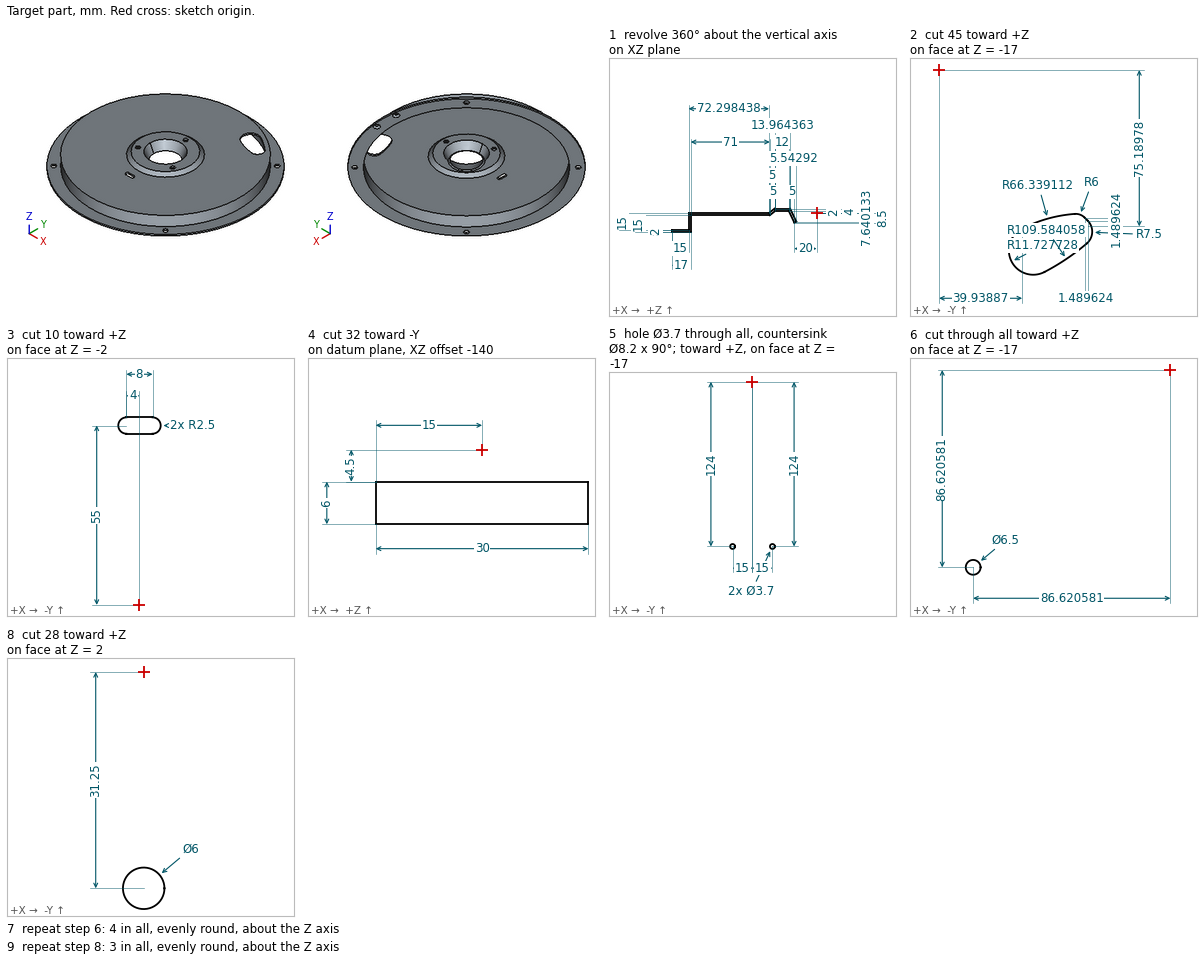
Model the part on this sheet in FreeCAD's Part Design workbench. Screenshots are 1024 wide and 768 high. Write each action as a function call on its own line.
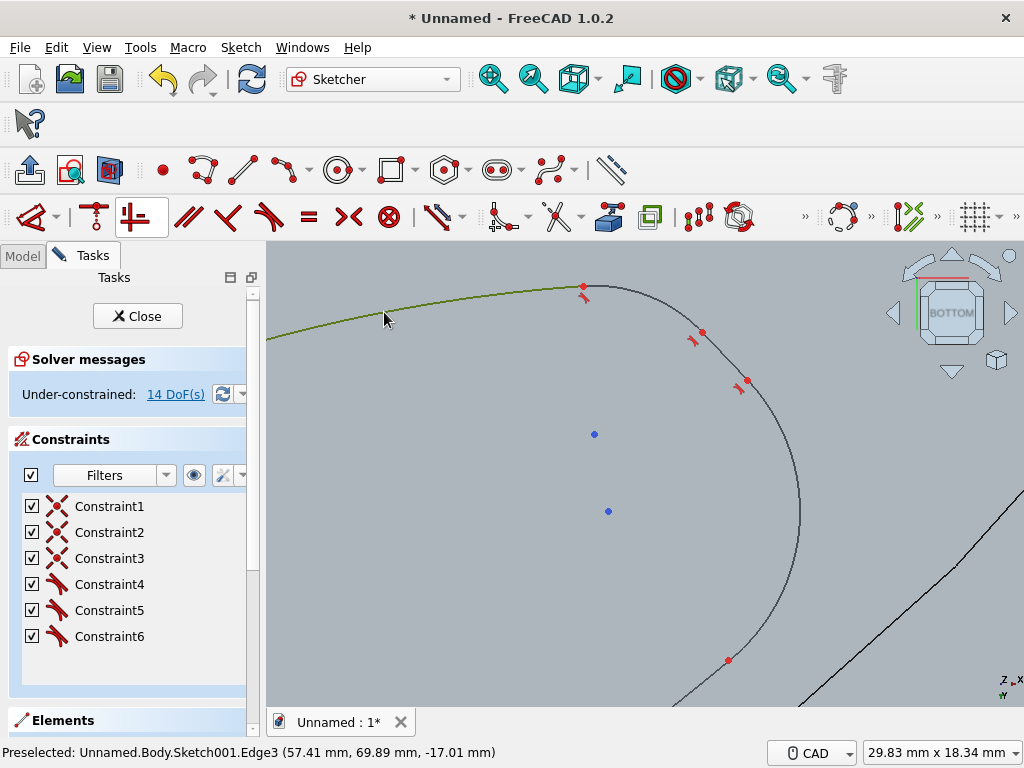
scroll(735, 372, down, 5)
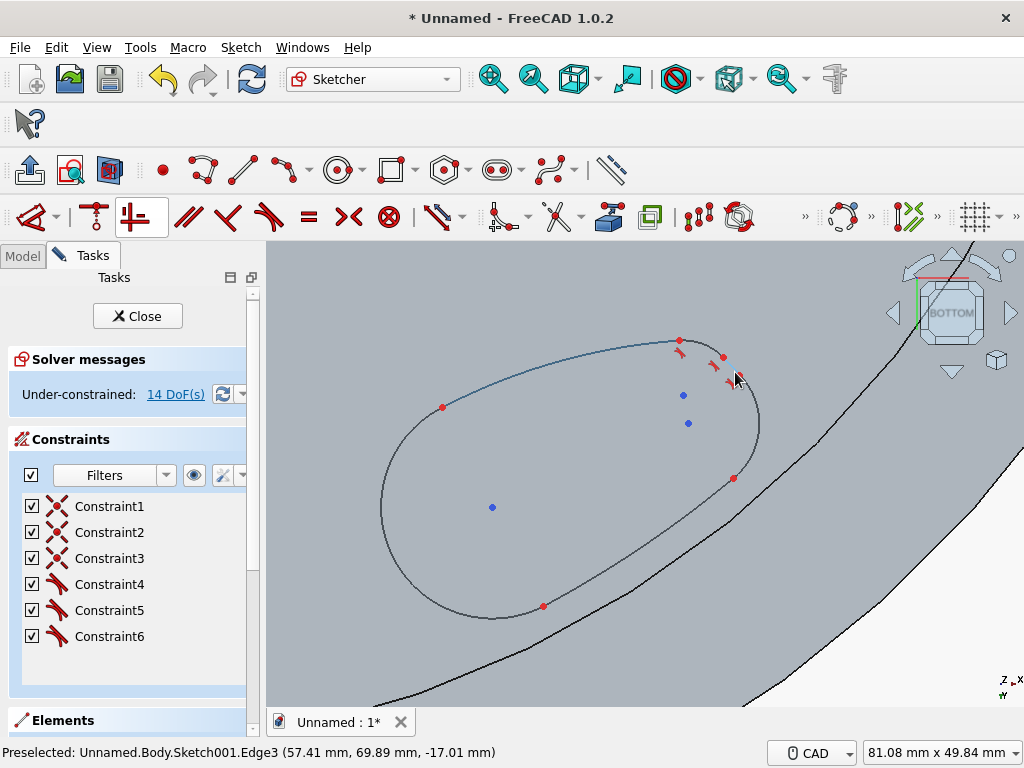
click(383, 489)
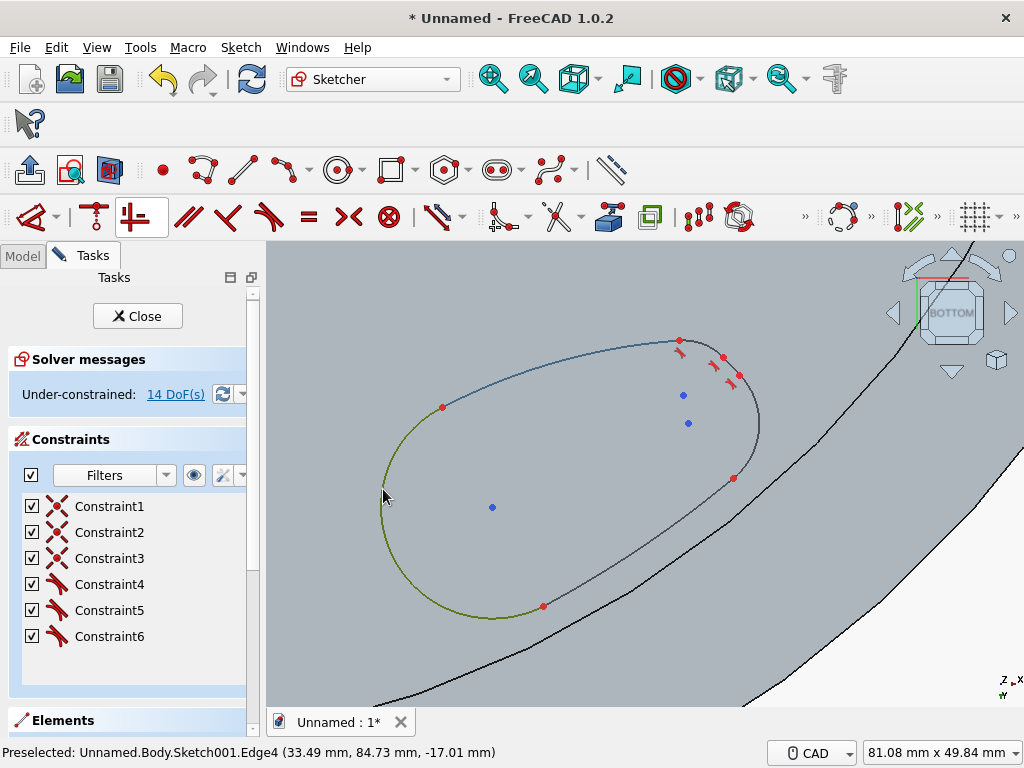
click(270, 218)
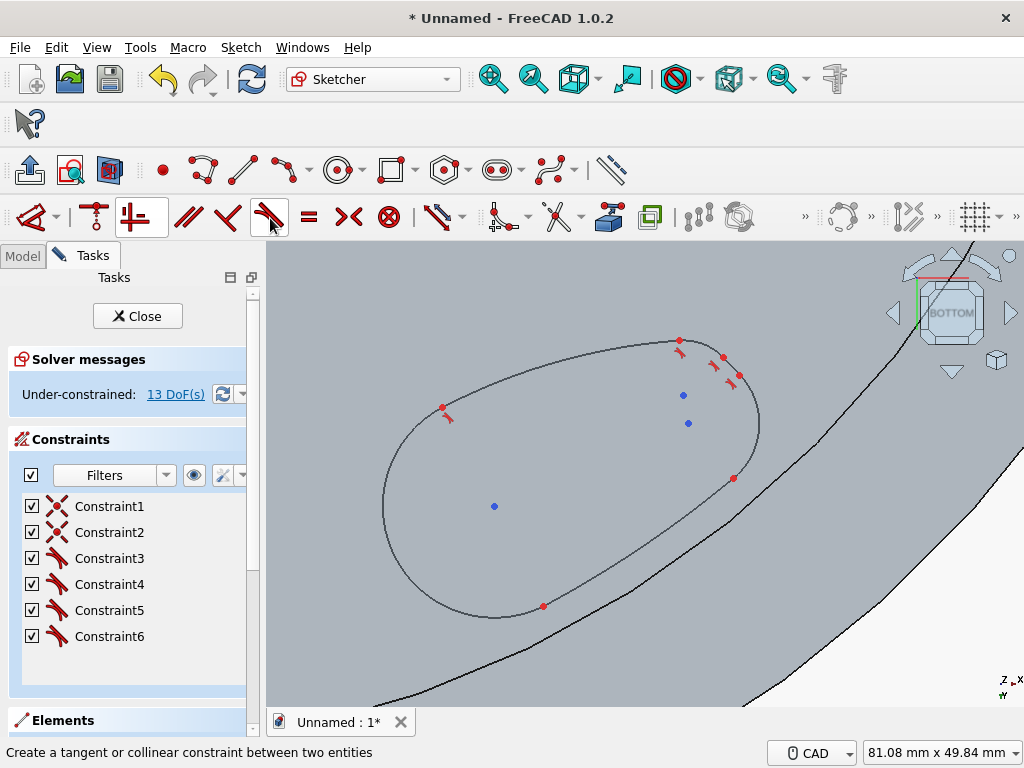
click(384, 489)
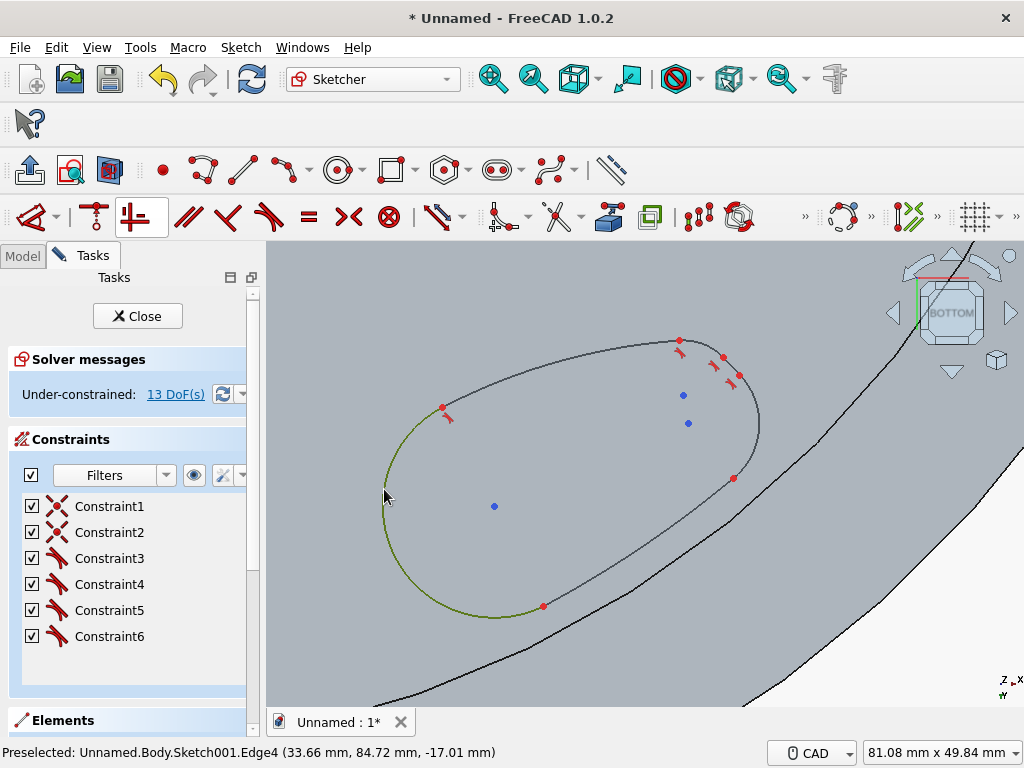
click(603, 572)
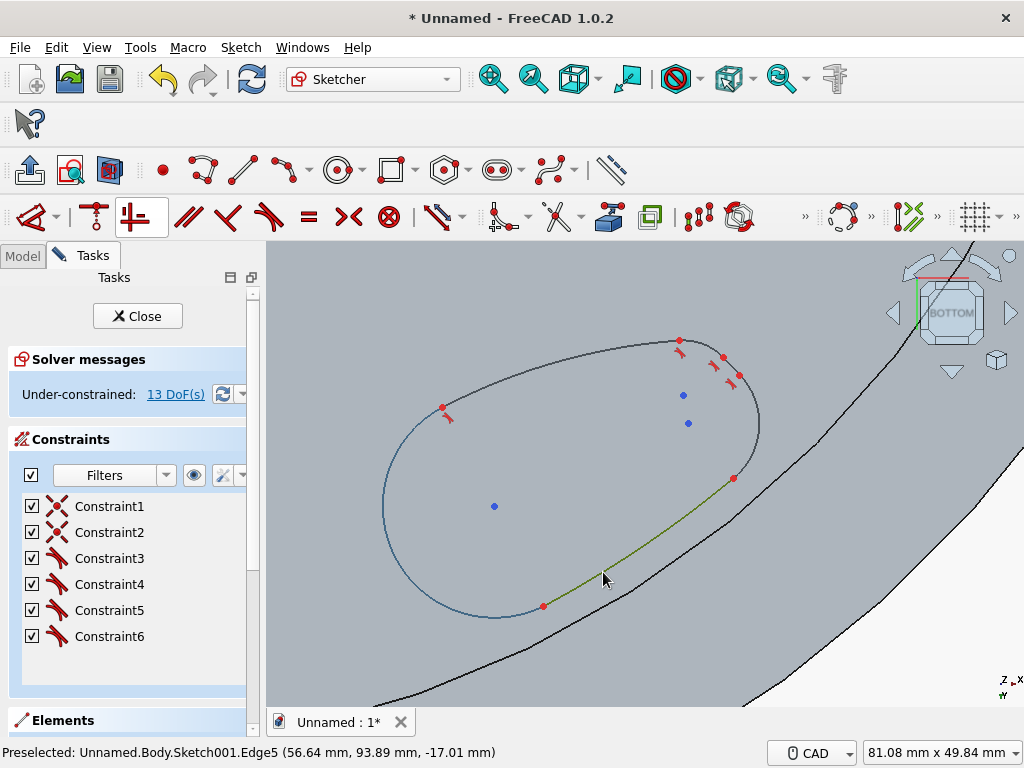
click(270, 218)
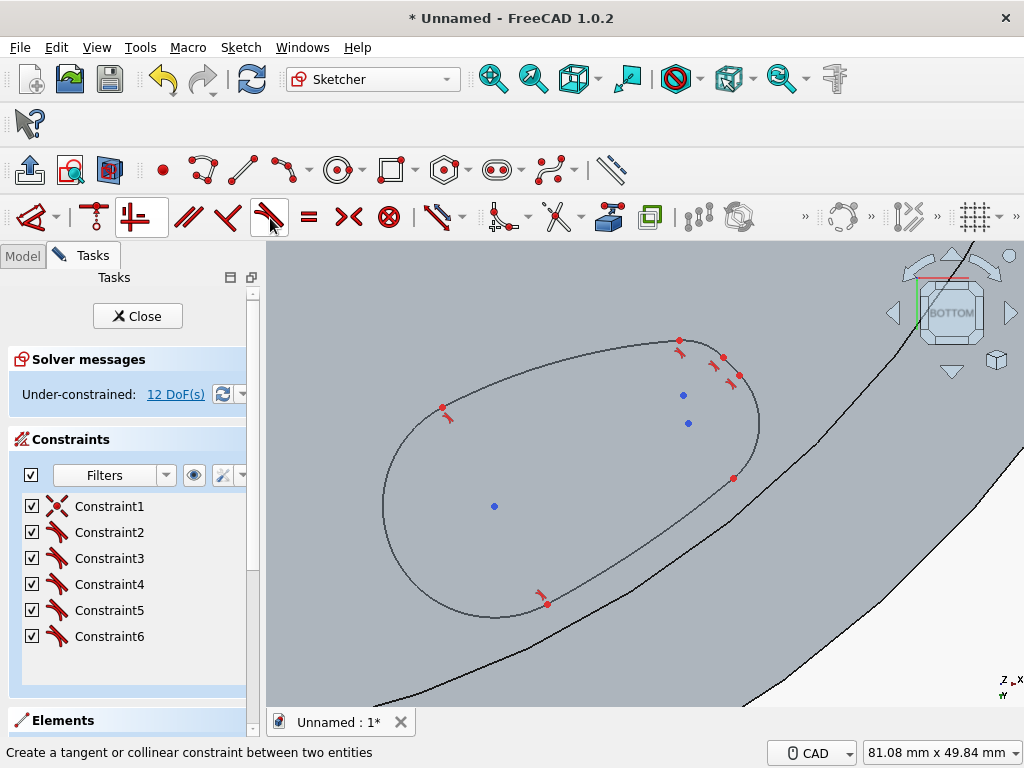
click(606, 570)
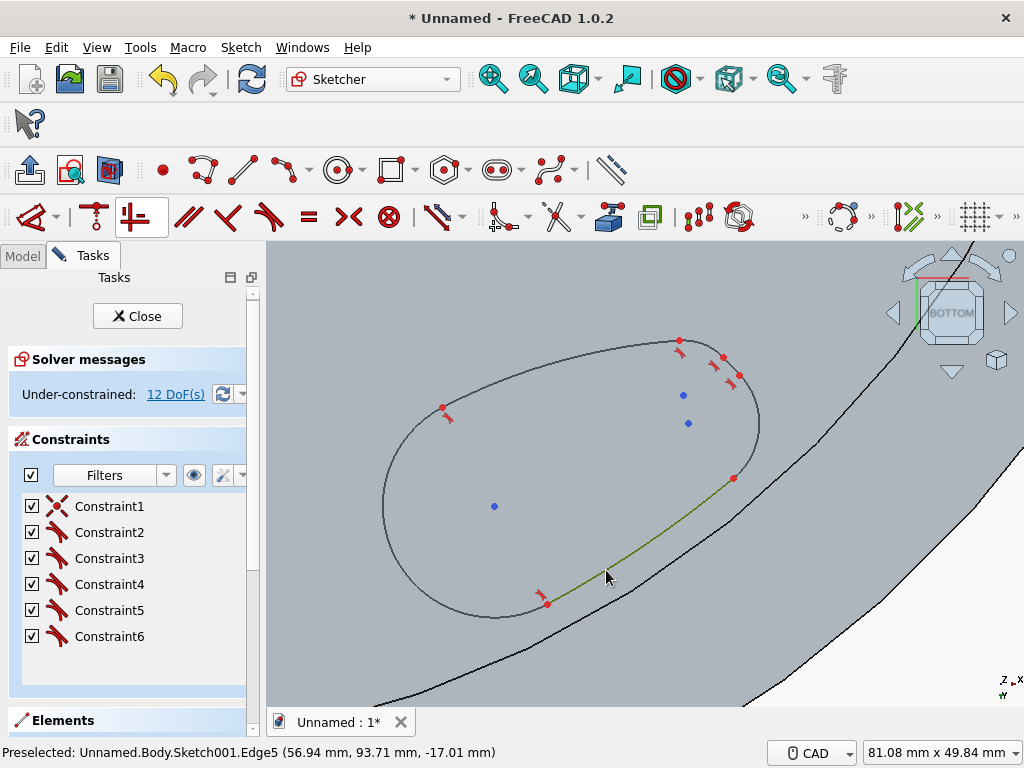
click(754, 451)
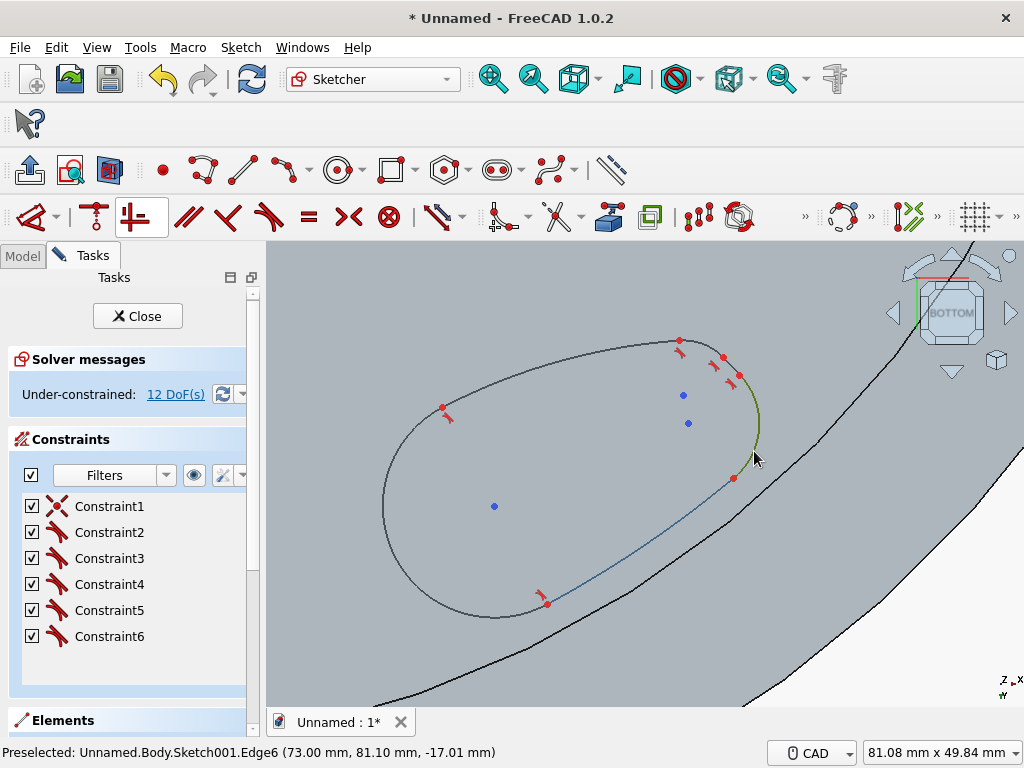
click(270, 218)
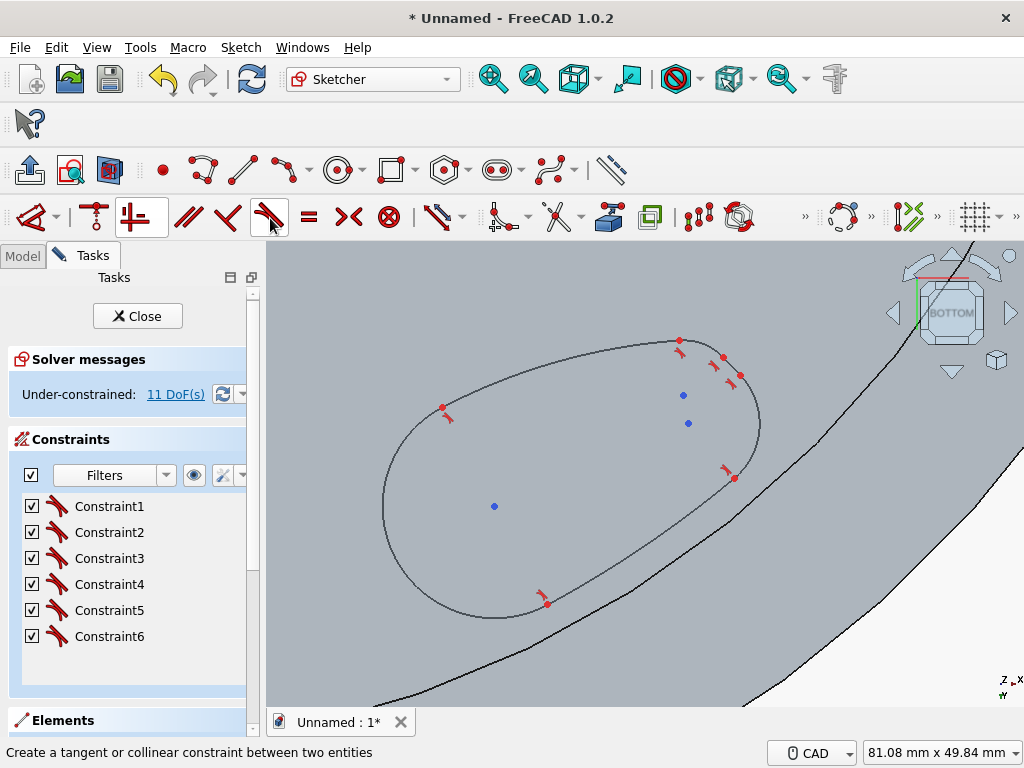
scroll(653, 622, down, 6)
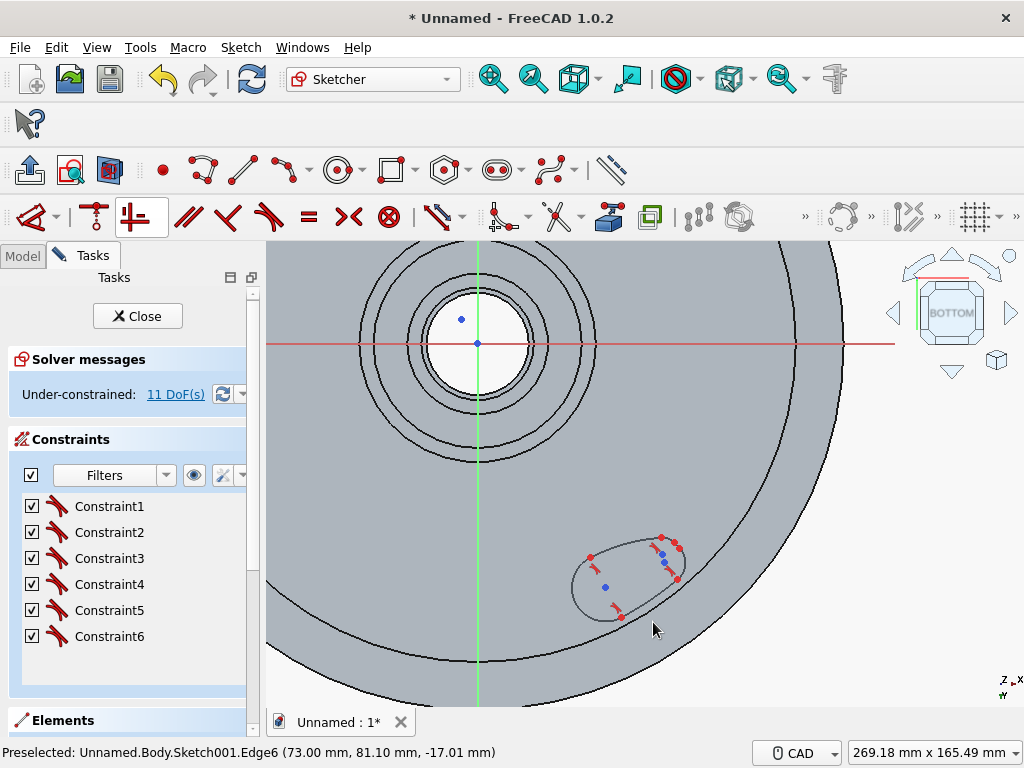
scroll(469, 332, up, 5)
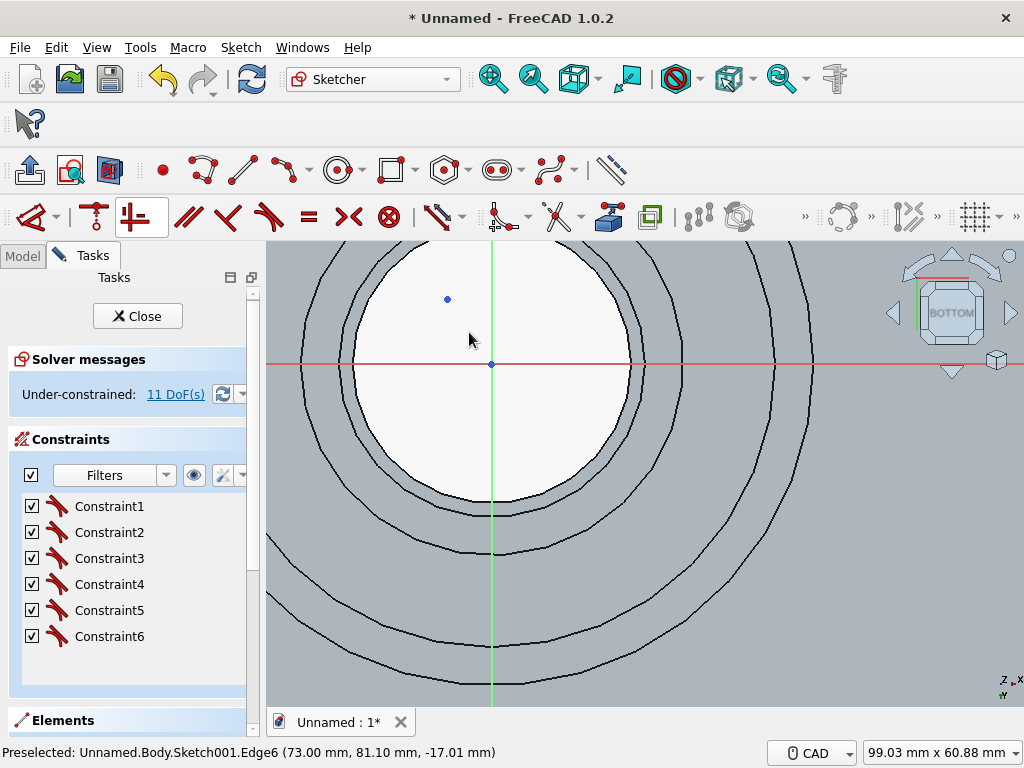
drag(437, 289, 502, 374)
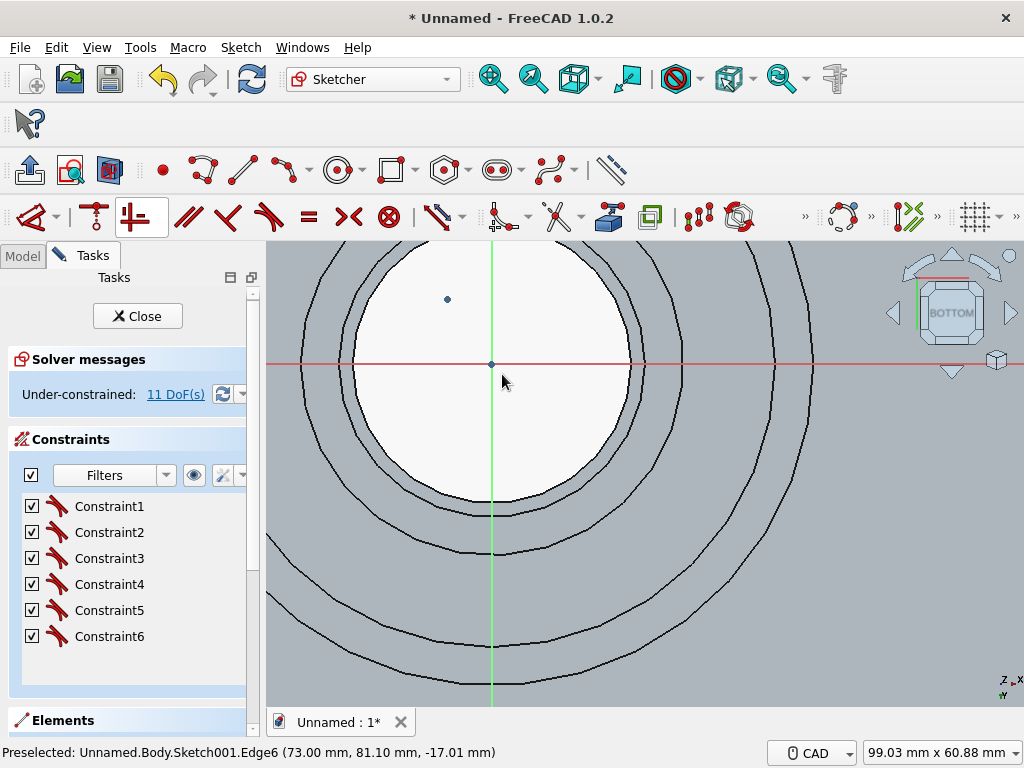
click(94, 218)